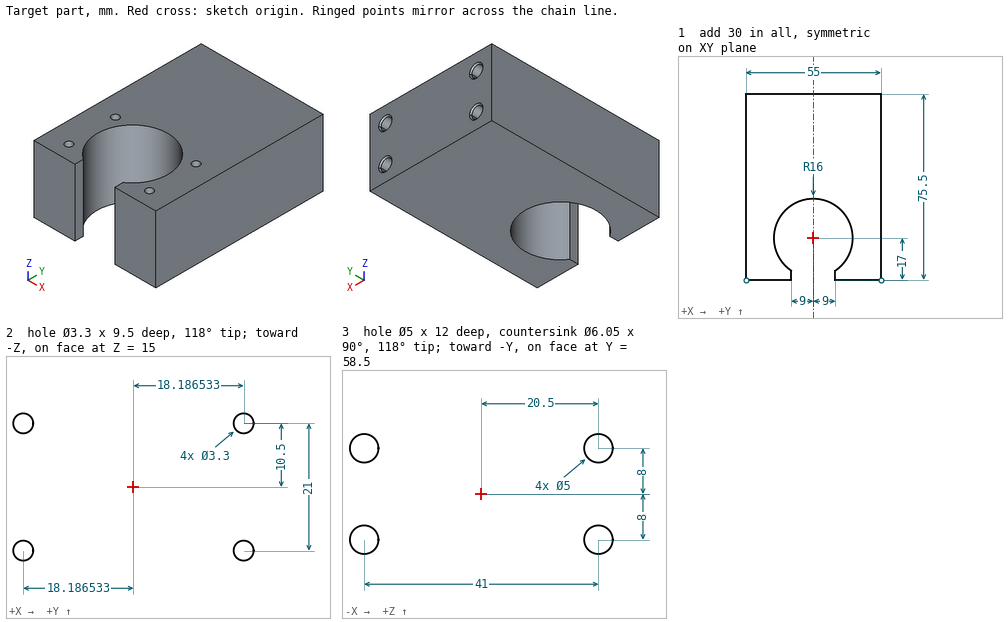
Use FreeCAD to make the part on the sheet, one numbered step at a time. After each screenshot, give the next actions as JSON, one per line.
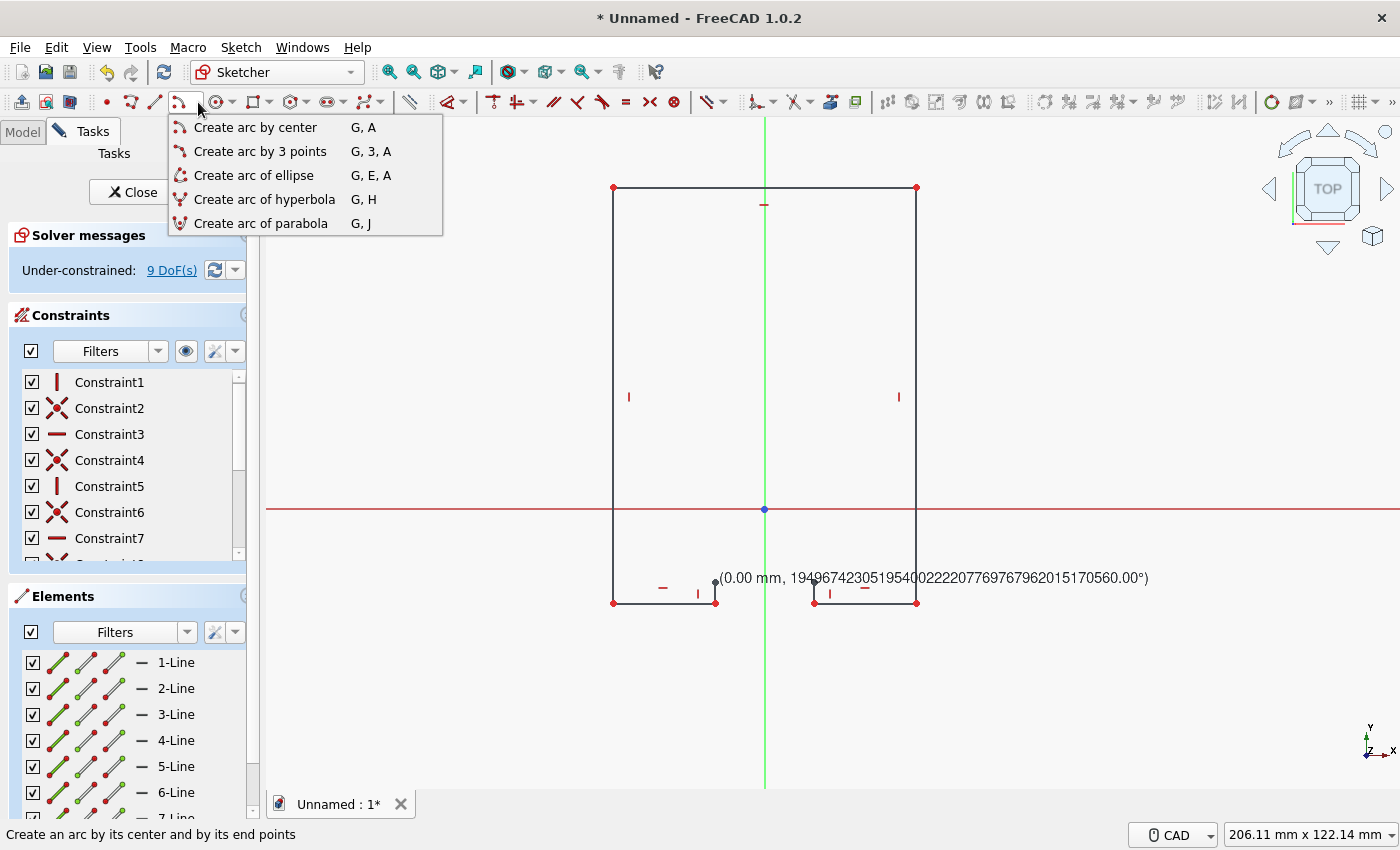
{"action": "left_click", "coordinate": [306, 151]}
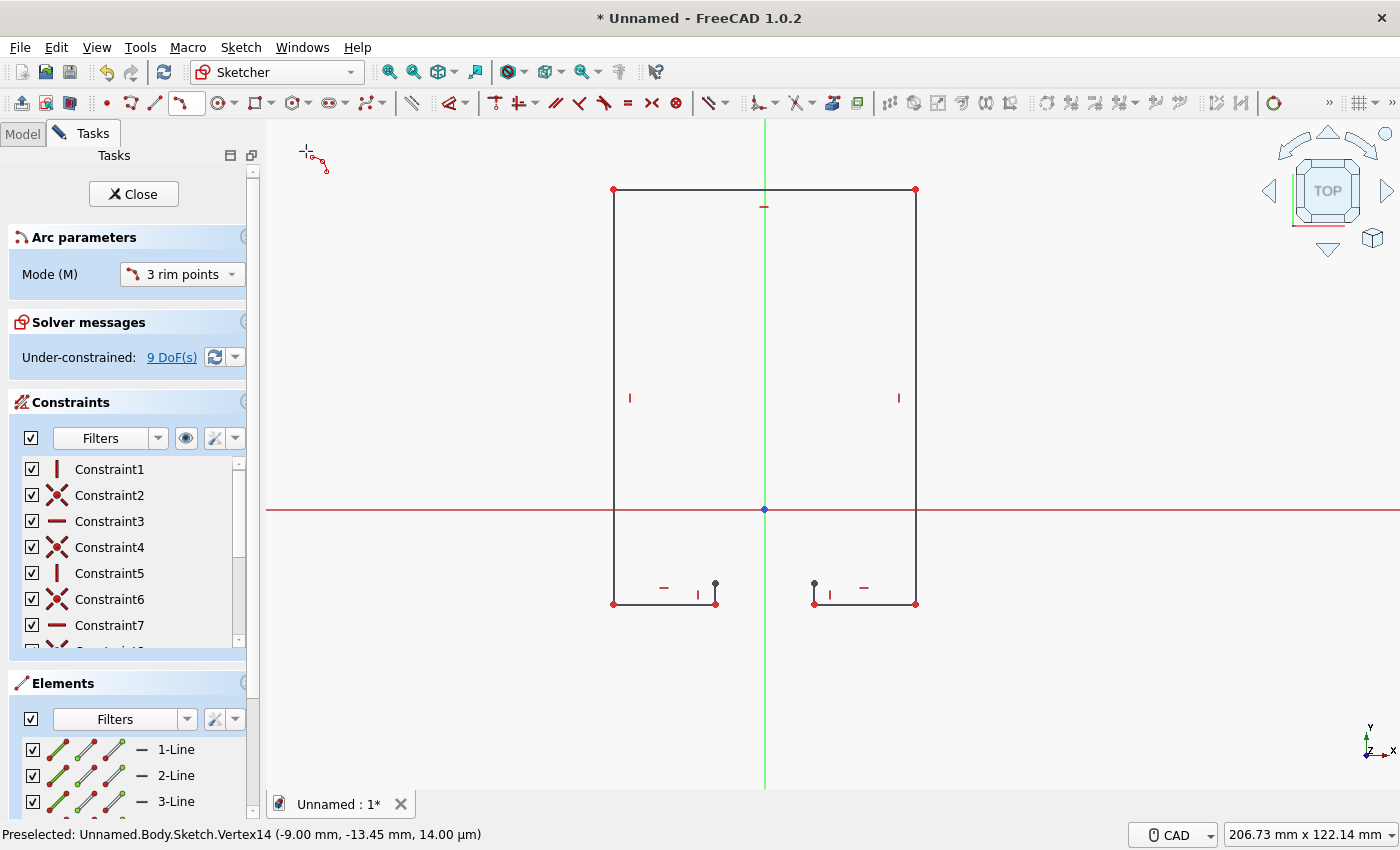
{"action": "scroll", "coordinate": [715, 582], "scroll_direction": "up", "scroll_amount": 3}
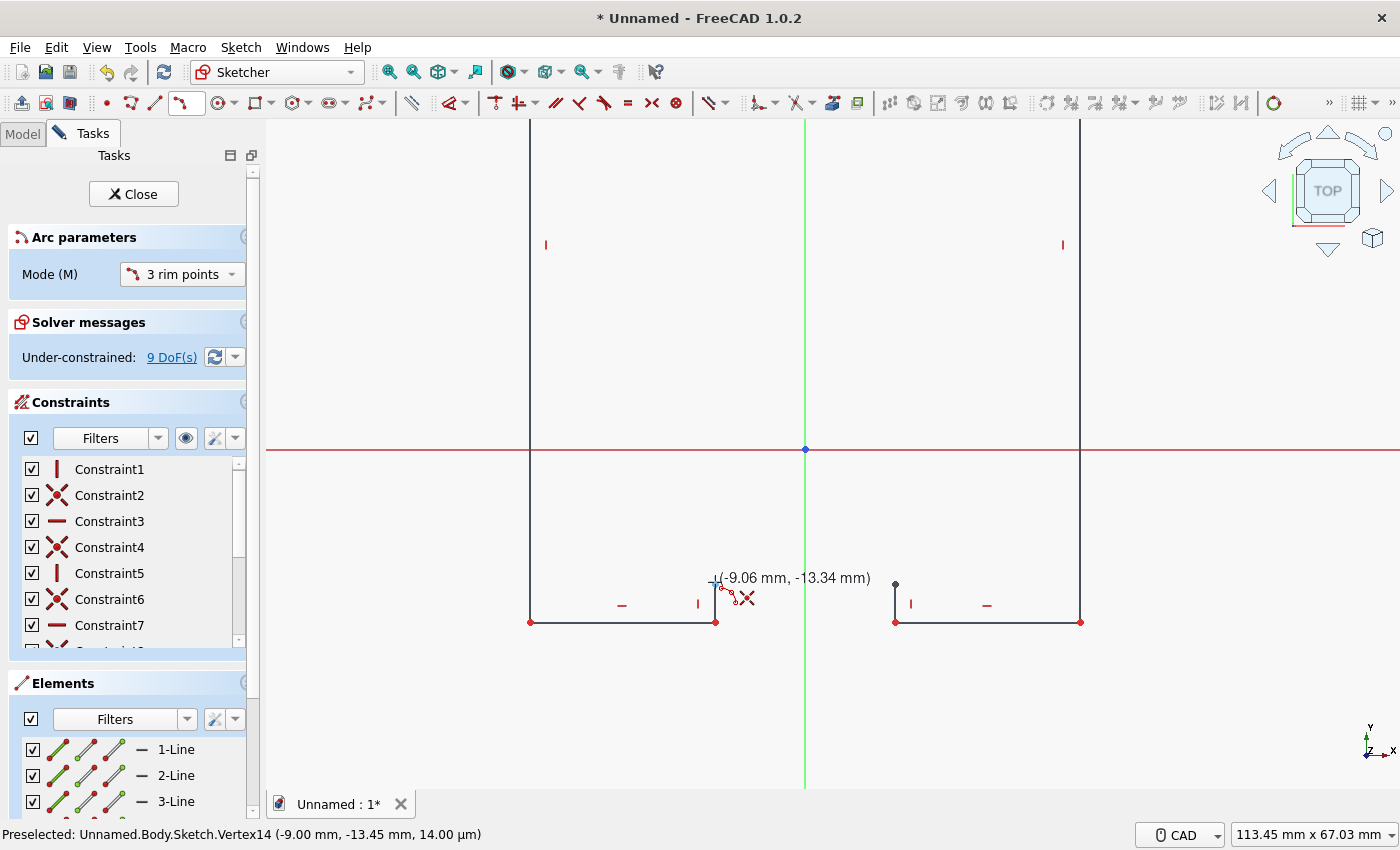
{"action": "left_click", "coordinate": [715, 584]}
{"action": "left_click", "coordinate": [895, 584]}
{"action": "left_click", "coordinate": [883, 310]}
{"action": "key", "text": "Escape"}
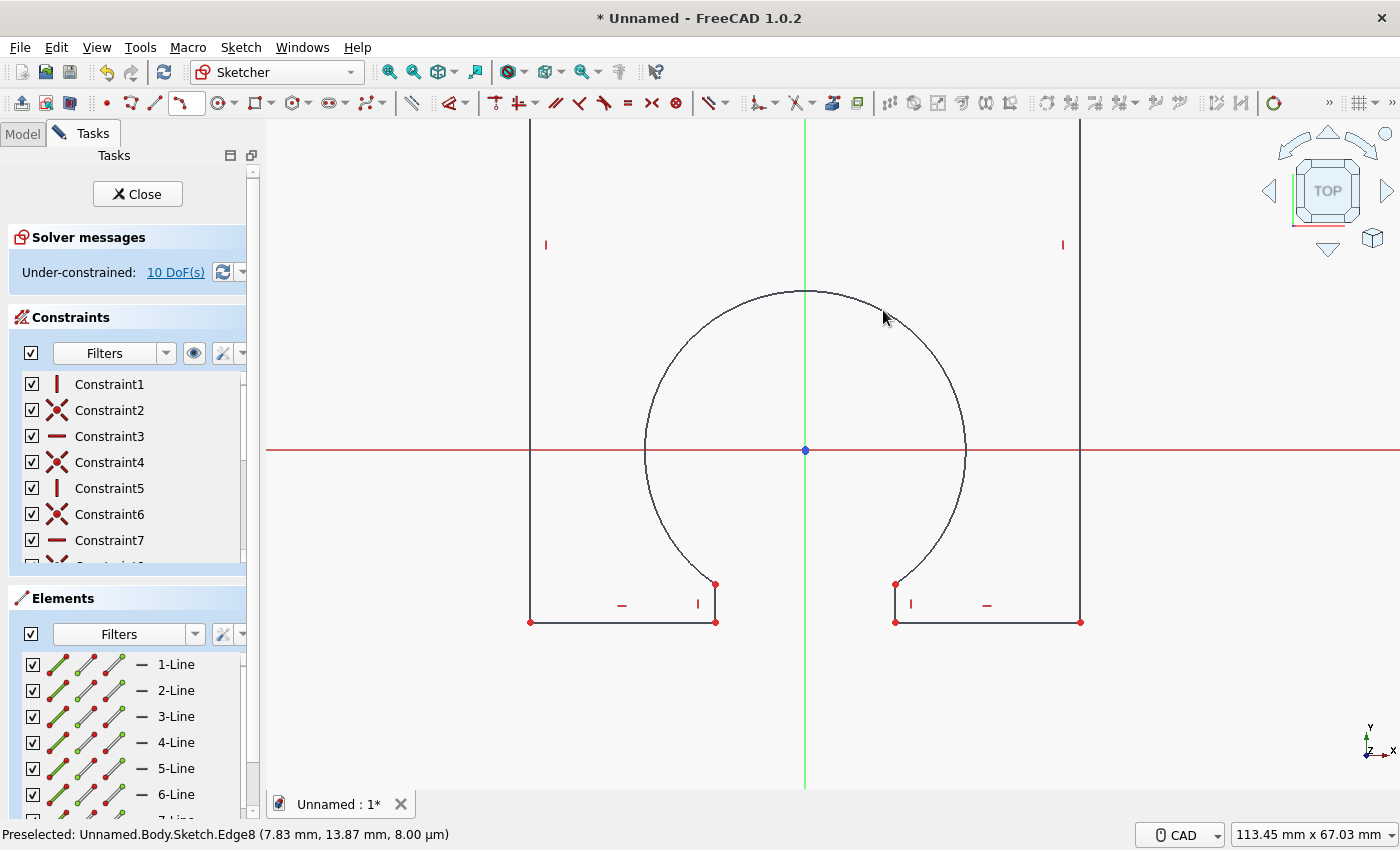
{"action": "left_click_drag", "start_coordinate": [795, 440], "coordinate": [815, 461]}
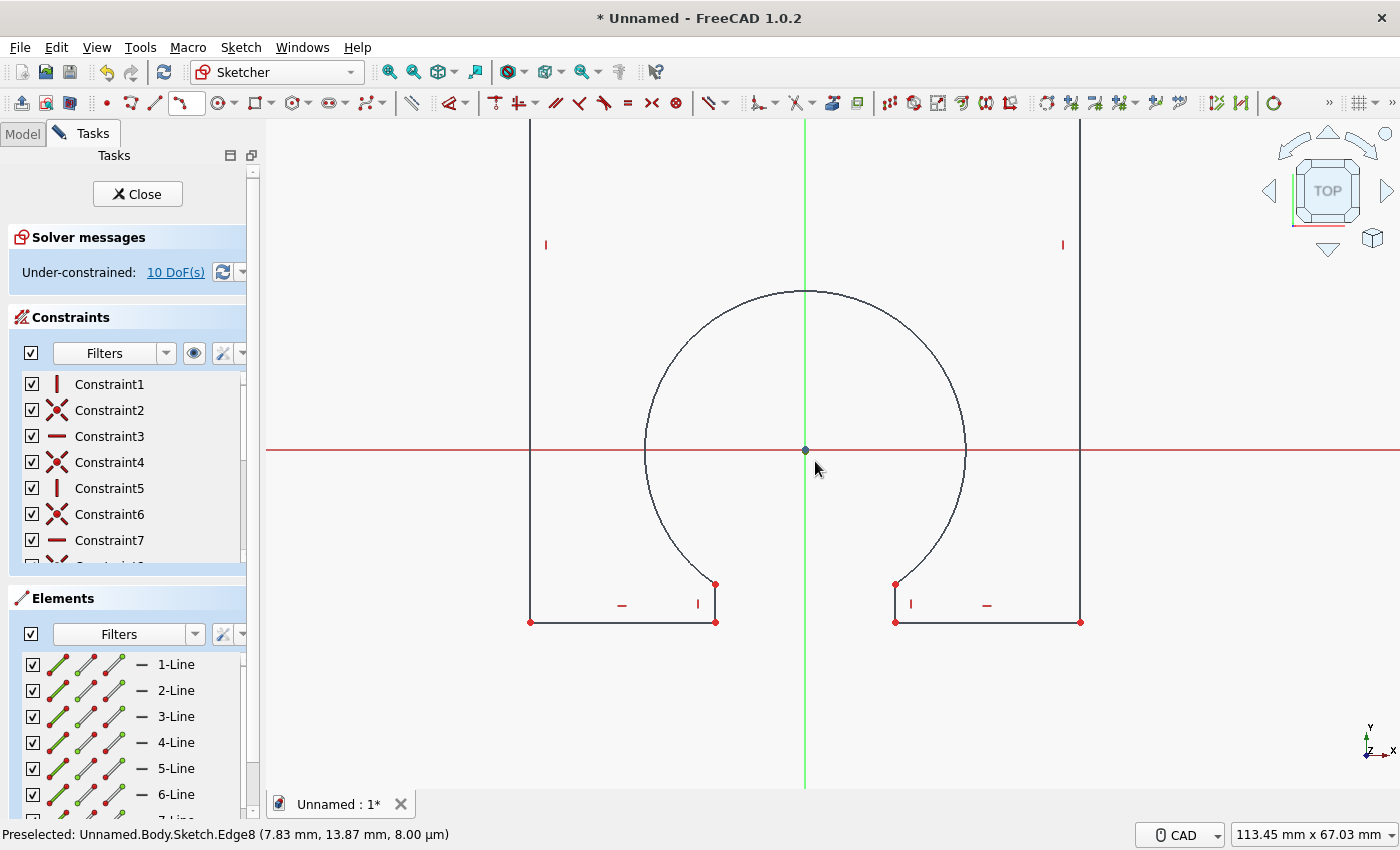
{"action": "left_click", "coordinate": [496, 104]}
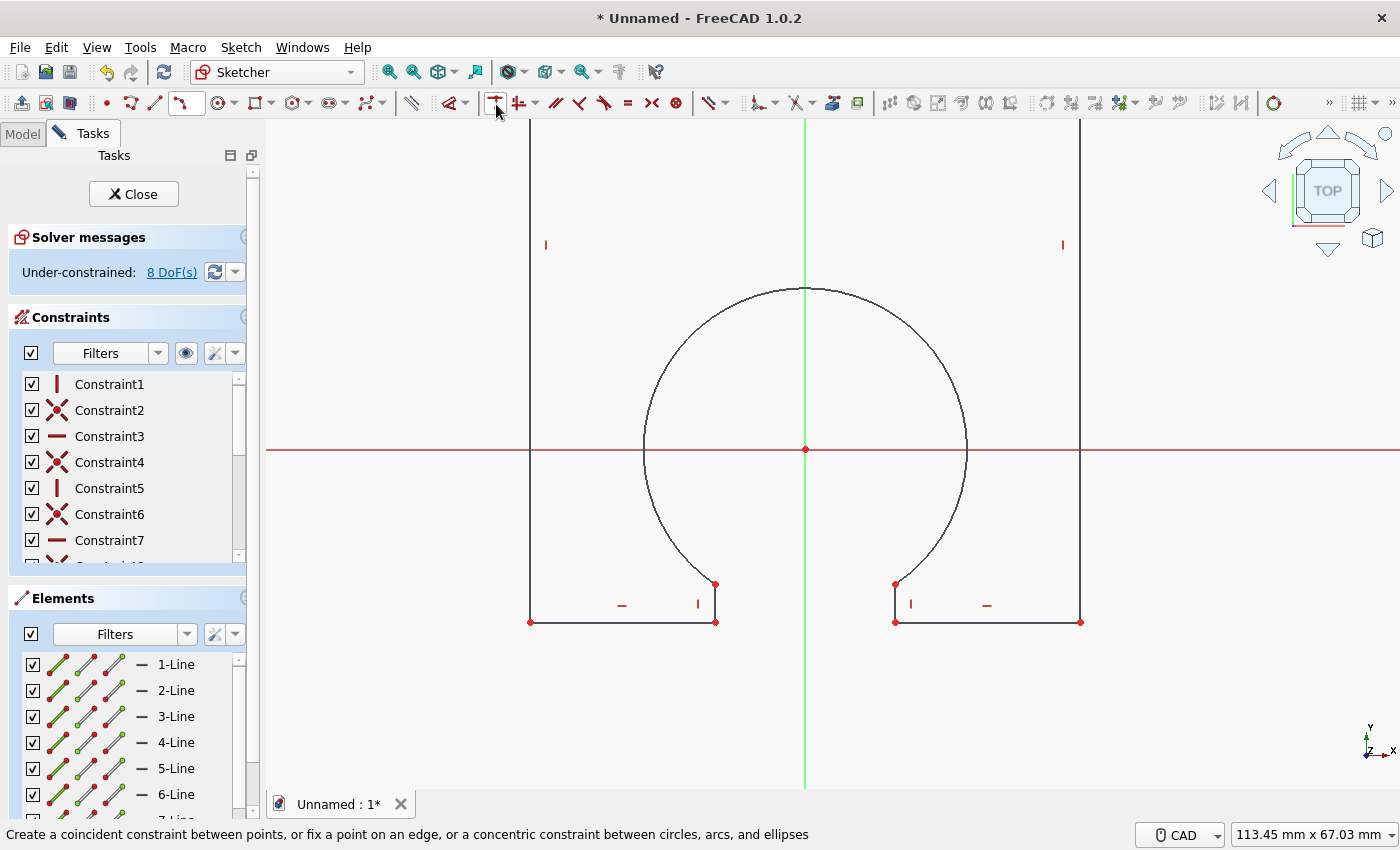
{"action": "left_click", "coordinate": [1080, 623]}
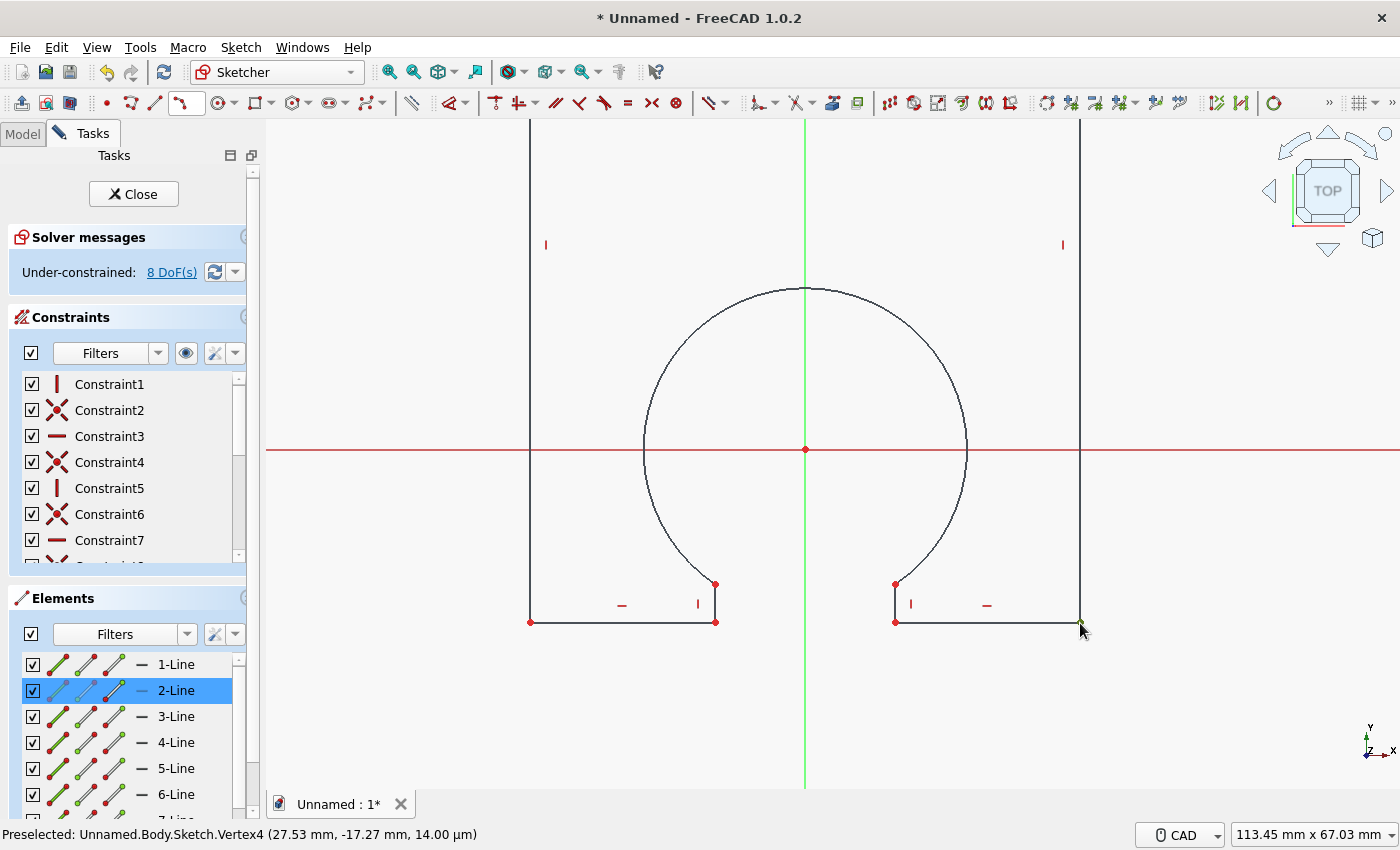
{"action": "left_click", "coordinate": [530, 623]}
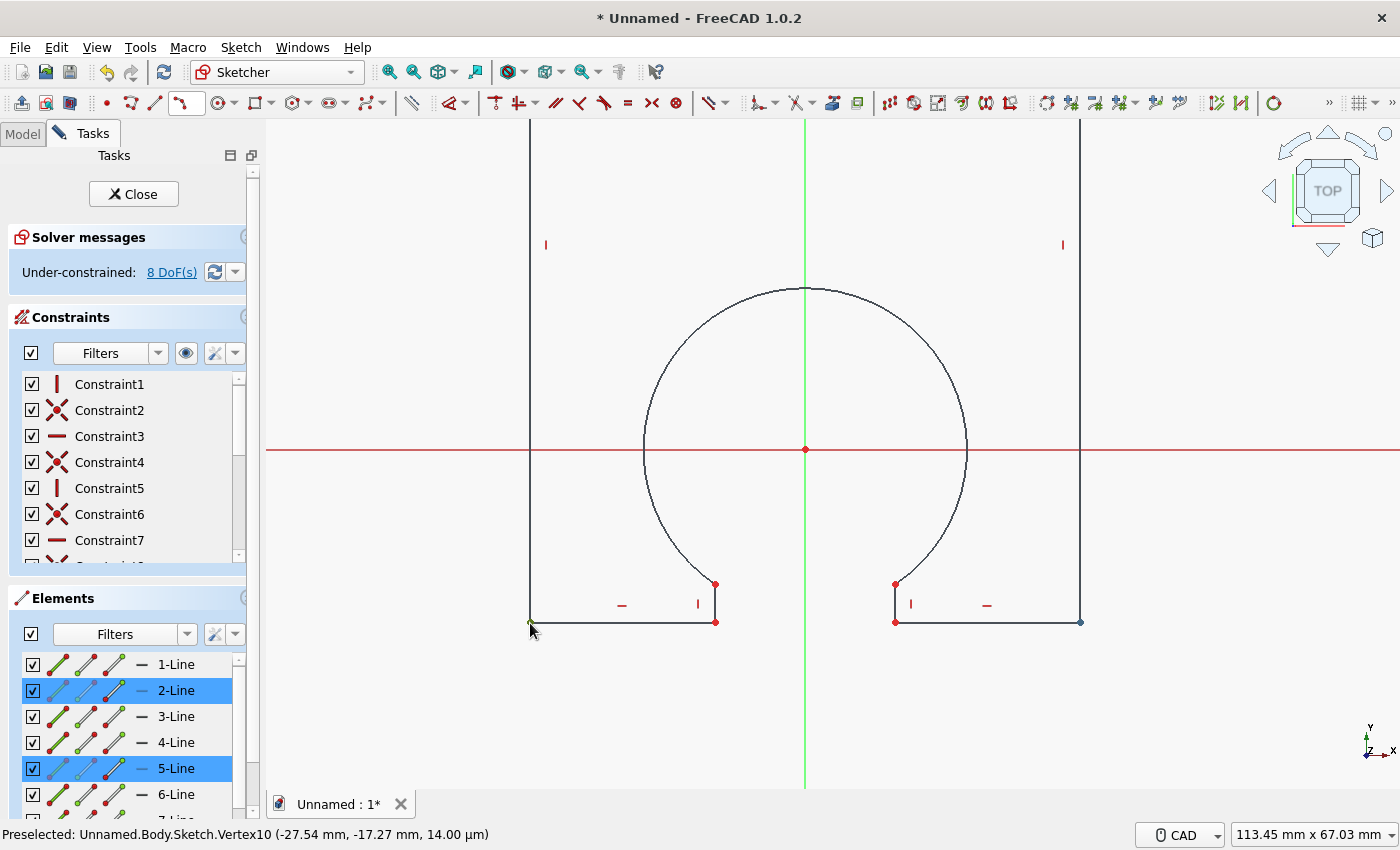
{"action": "left_click", "coordinate": [805, 717]}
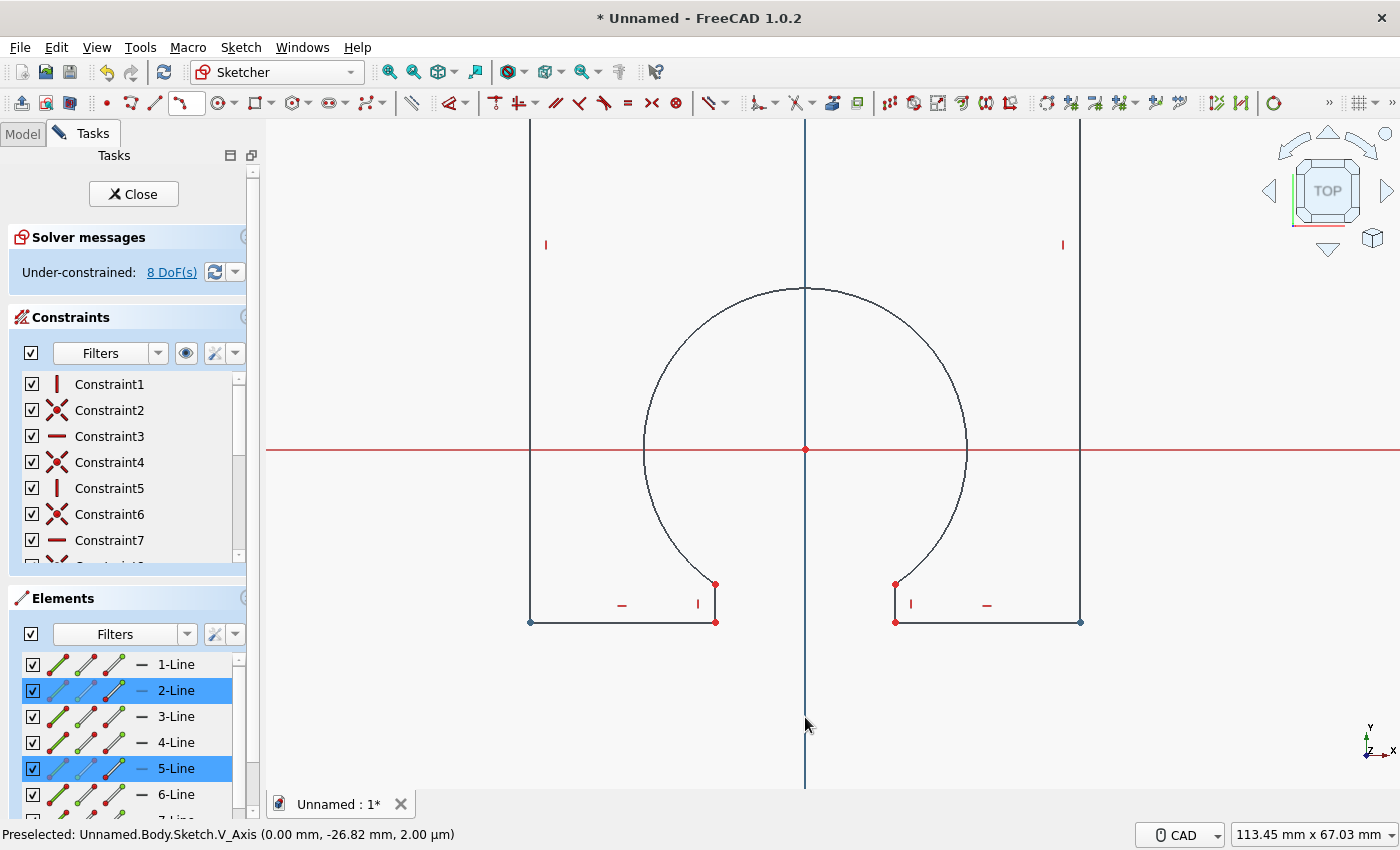
{"action": "left_click", "coordinate": [652, 104]}